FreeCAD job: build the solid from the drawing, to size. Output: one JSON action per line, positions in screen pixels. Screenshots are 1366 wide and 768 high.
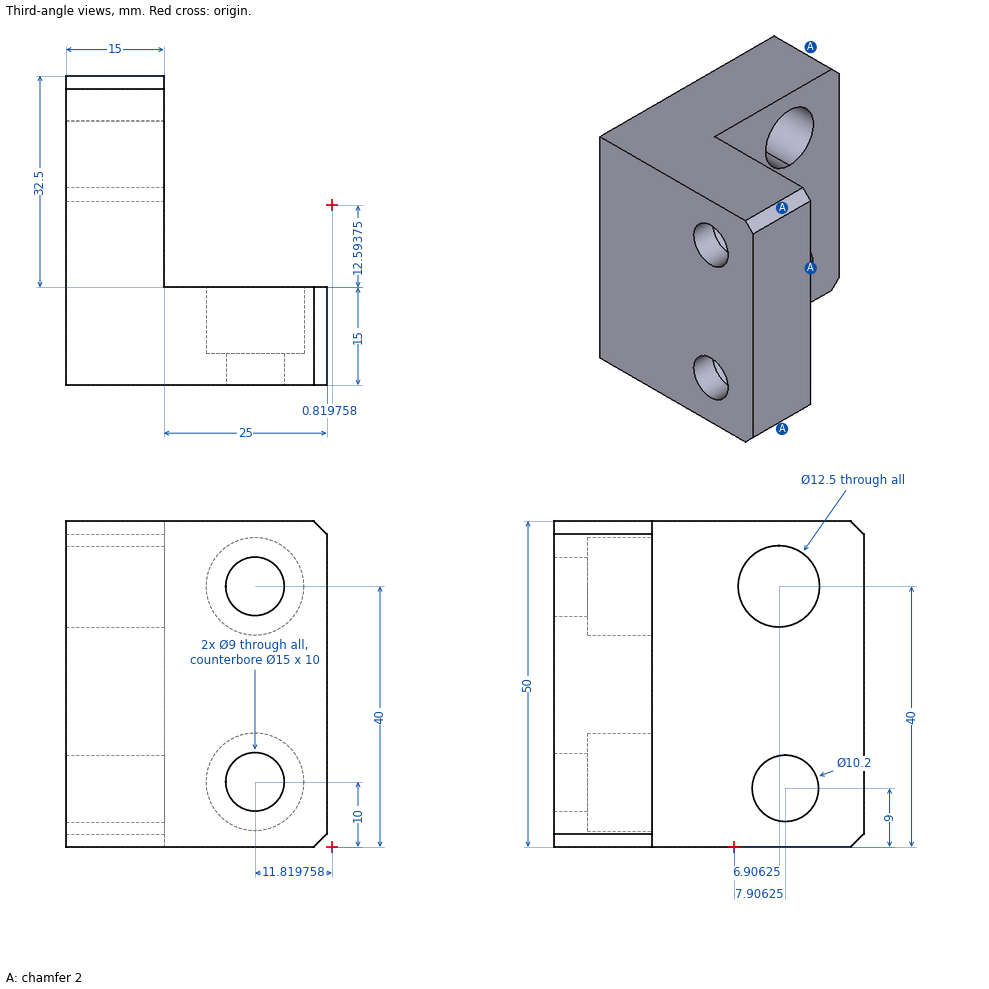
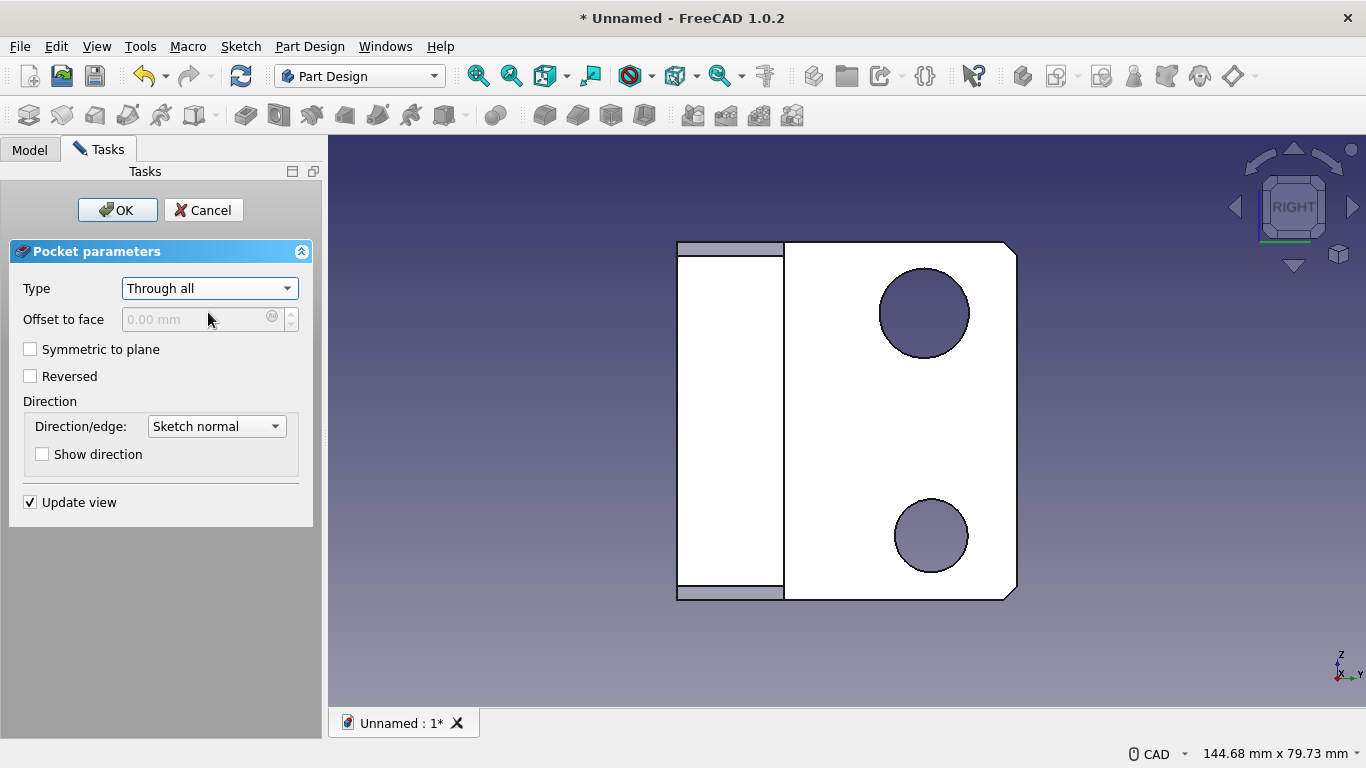
{"action": "left_click", "coordinate": [118, 210]}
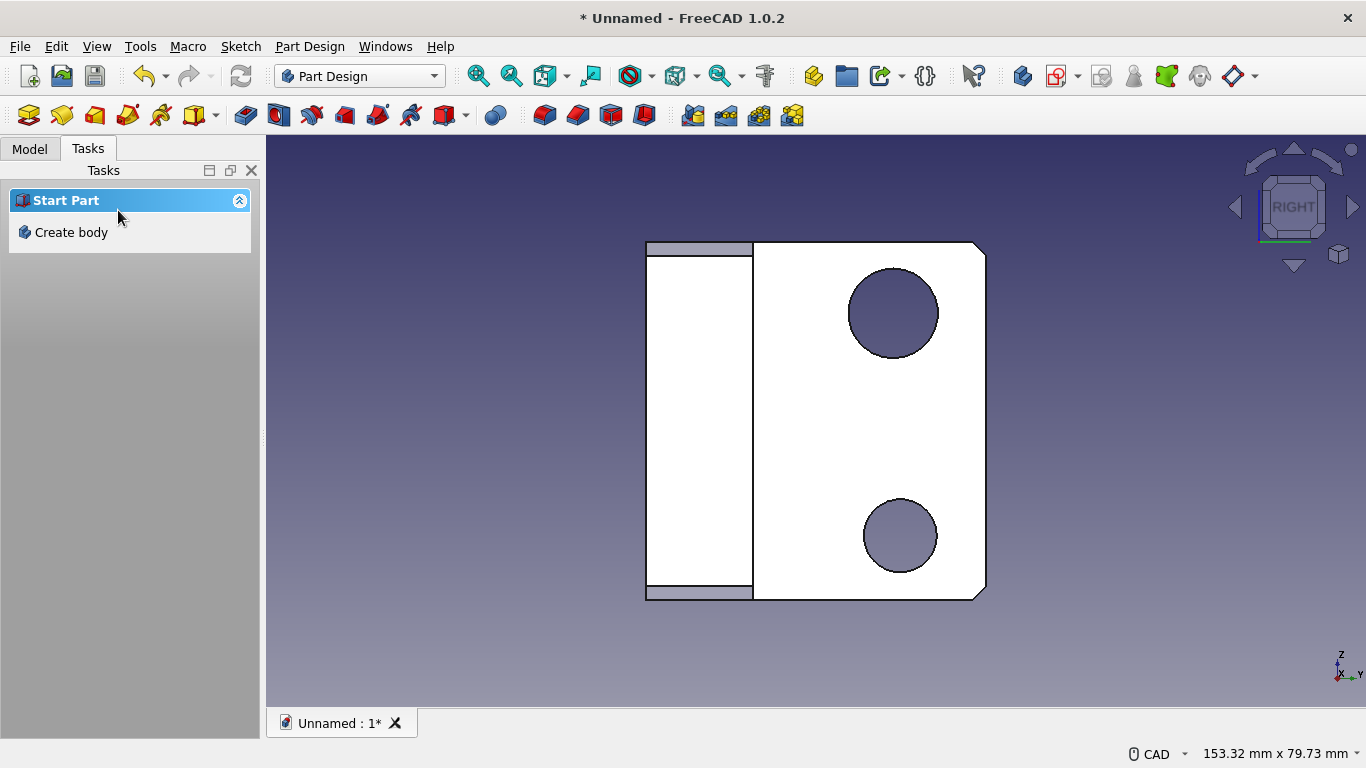
{"action": "key", "text": "0"}